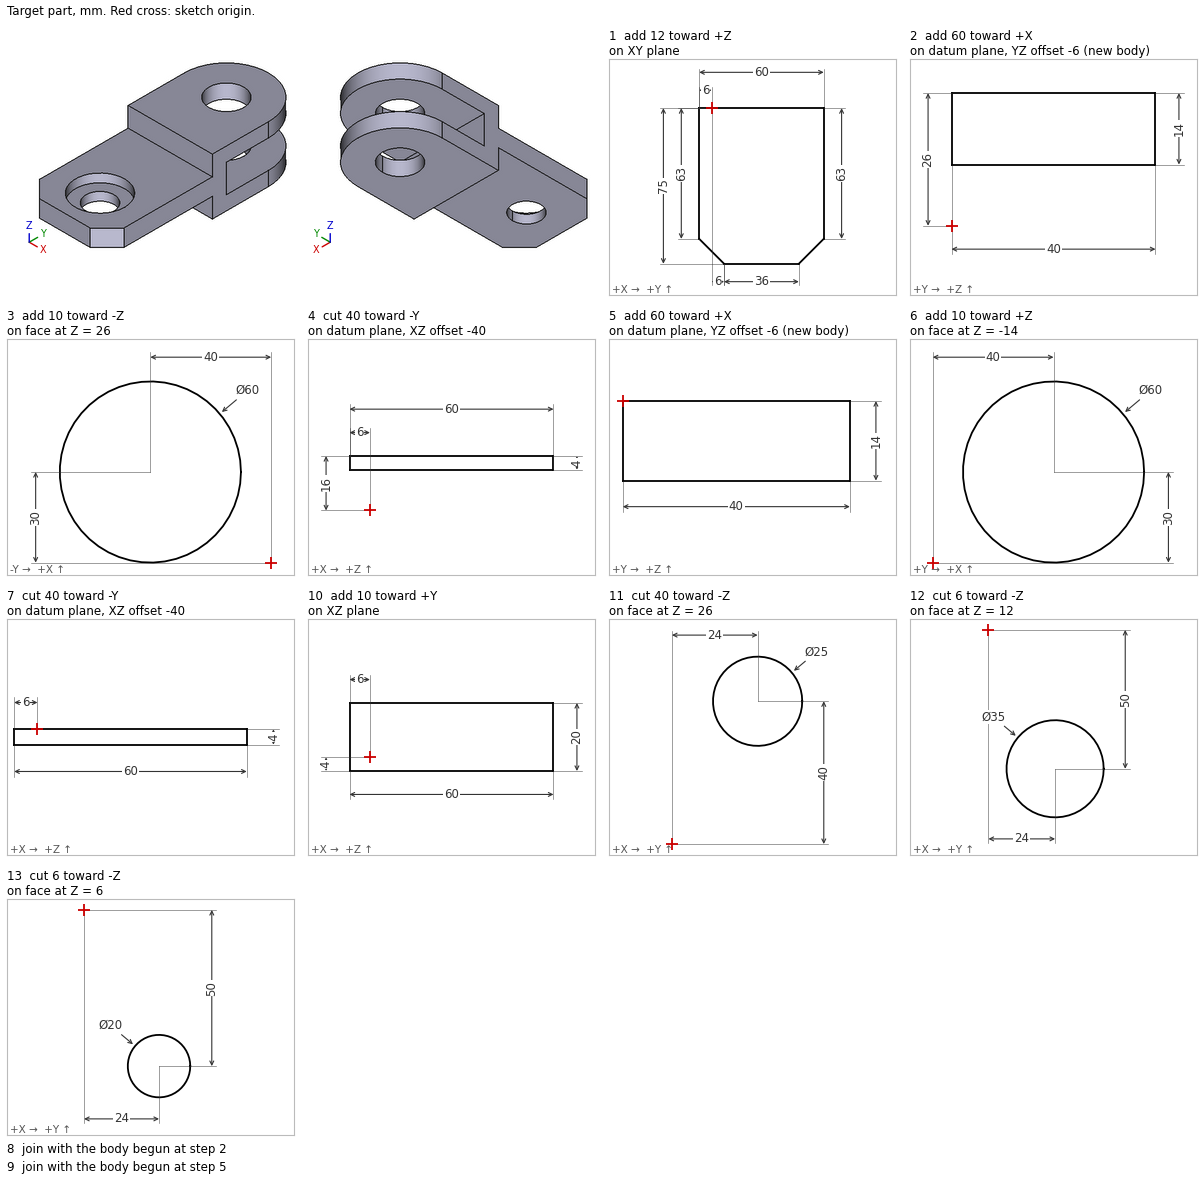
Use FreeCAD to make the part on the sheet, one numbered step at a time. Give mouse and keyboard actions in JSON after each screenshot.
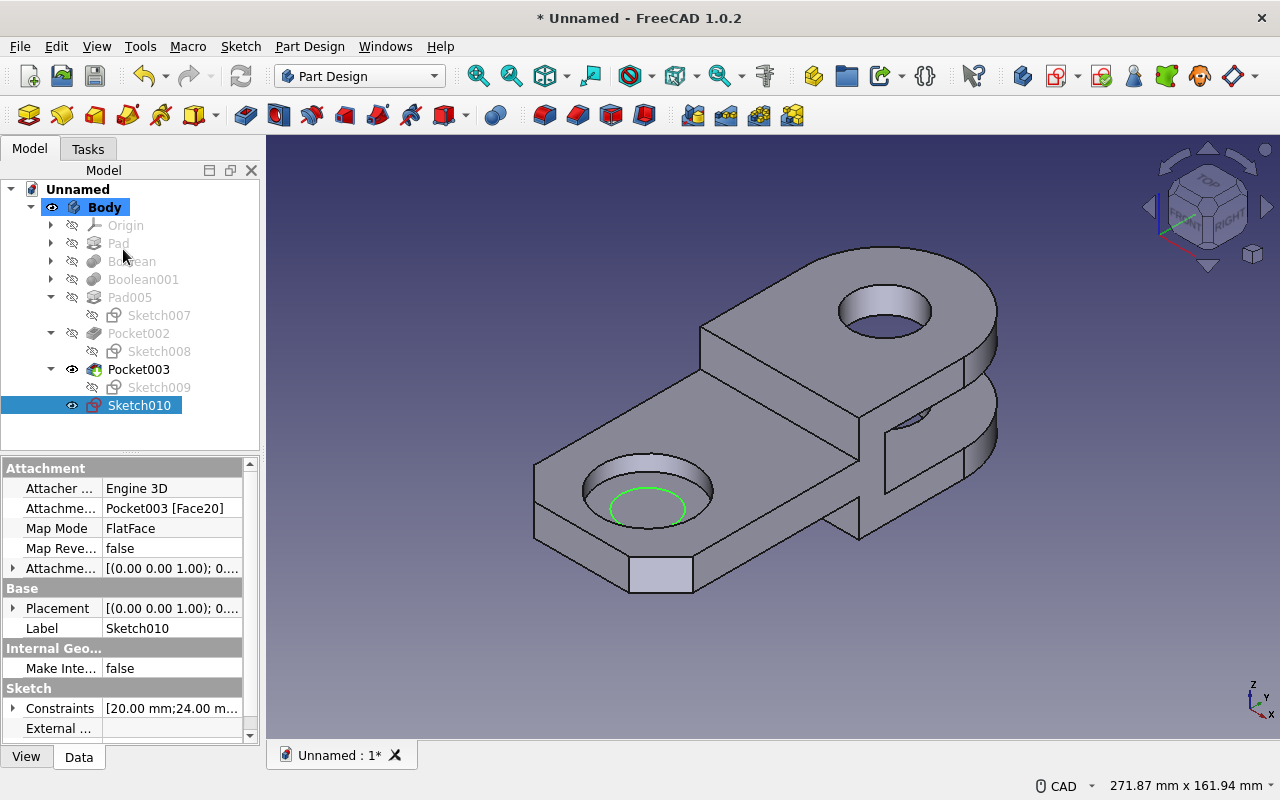
{"action": "left_click", "coordinate": [246, 116]}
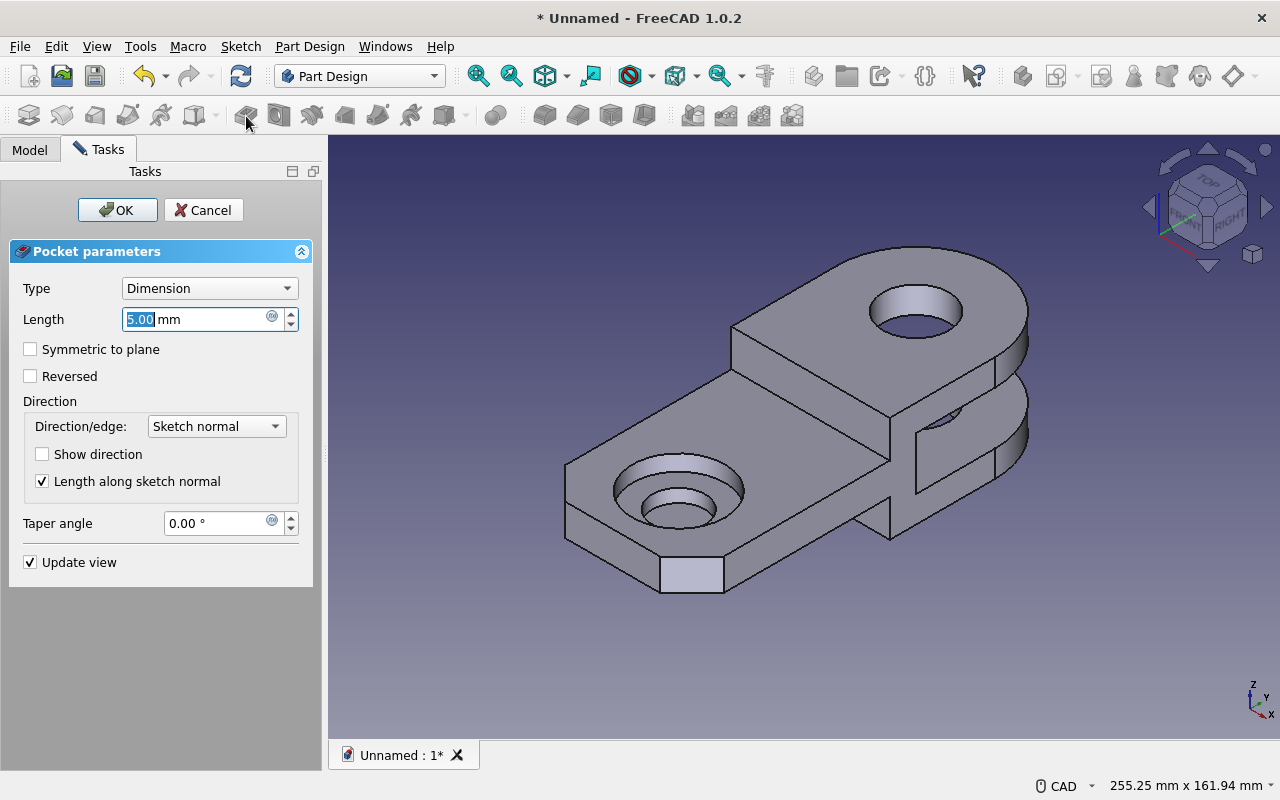
{"action": "type", "text": "6"}
{"action": "key", "text": "Tab"}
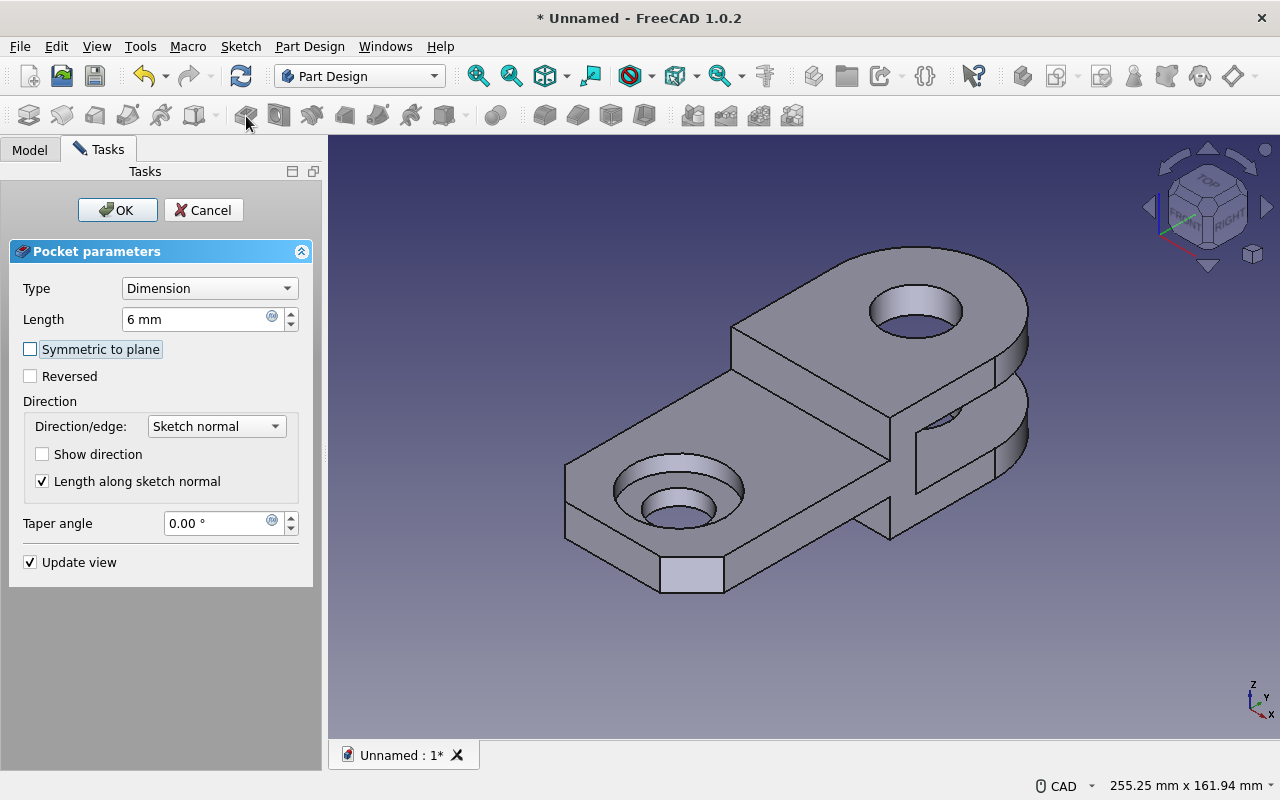
{"action": "left_click", "coordinate": [118, 210]}